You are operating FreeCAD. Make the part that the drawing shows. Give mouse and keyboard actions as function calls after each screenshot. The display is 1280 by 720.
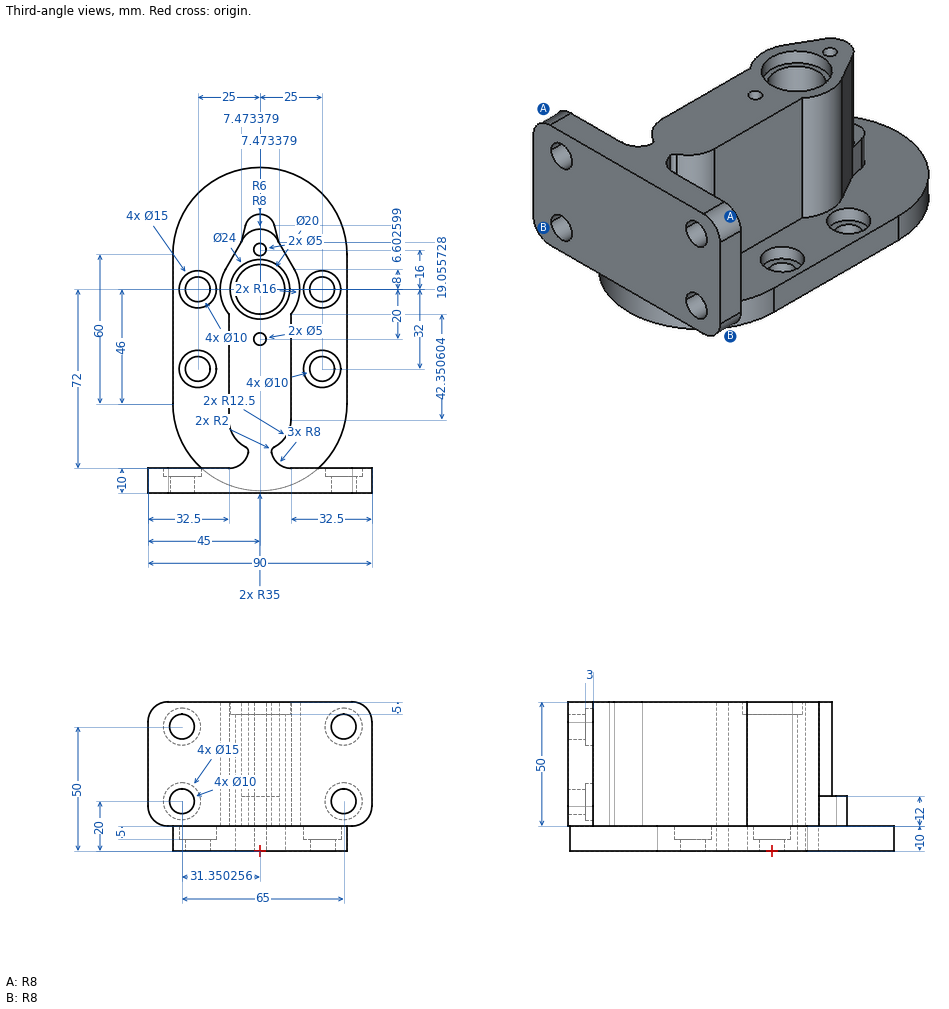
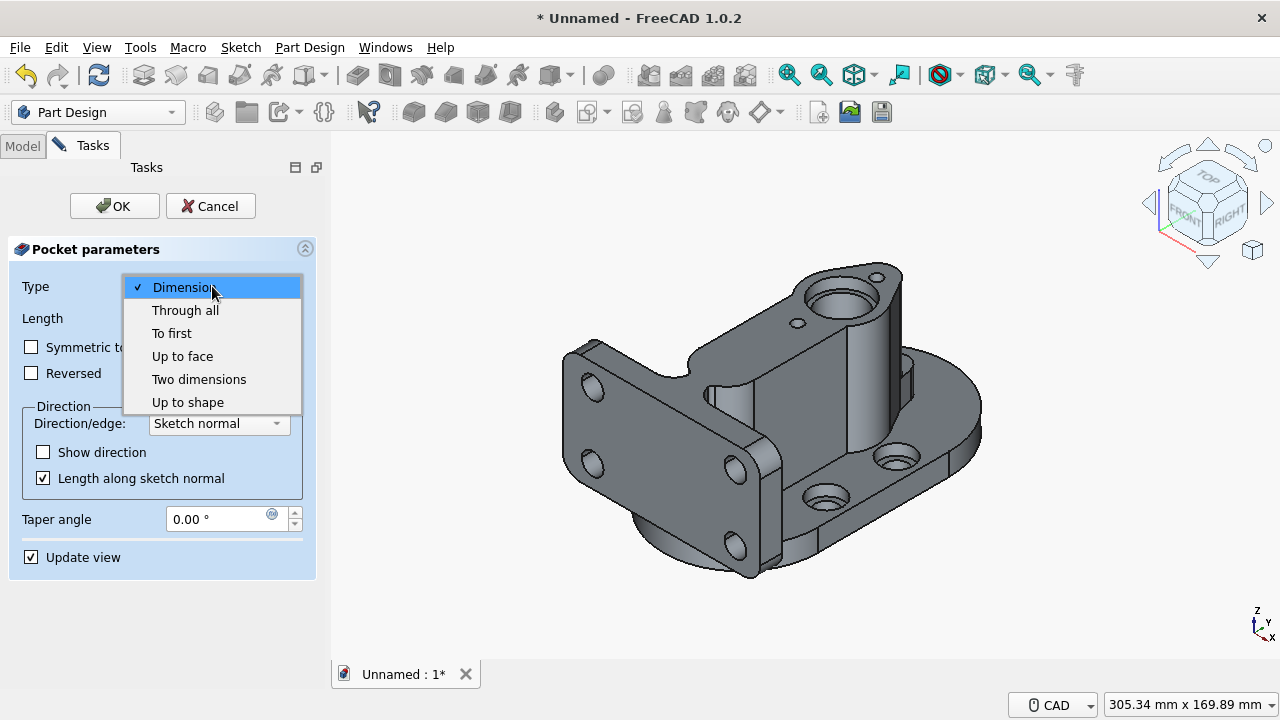
click(212, 310)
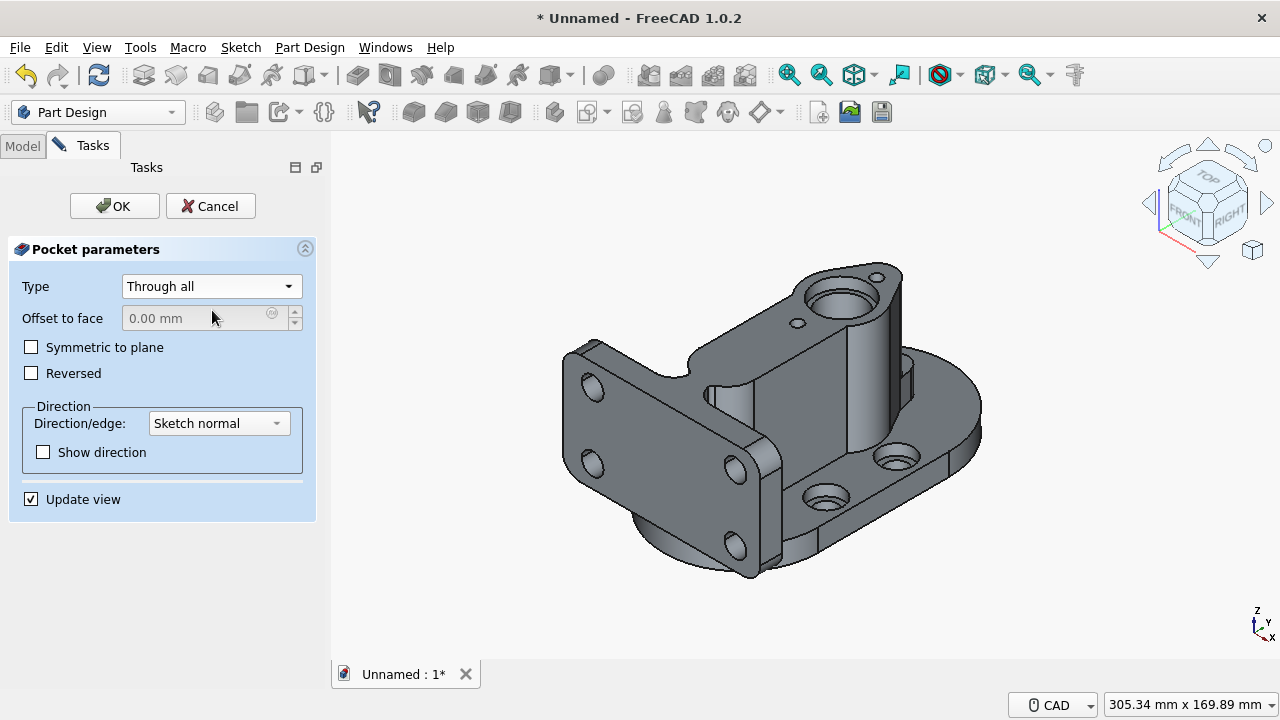
click(115, 206)